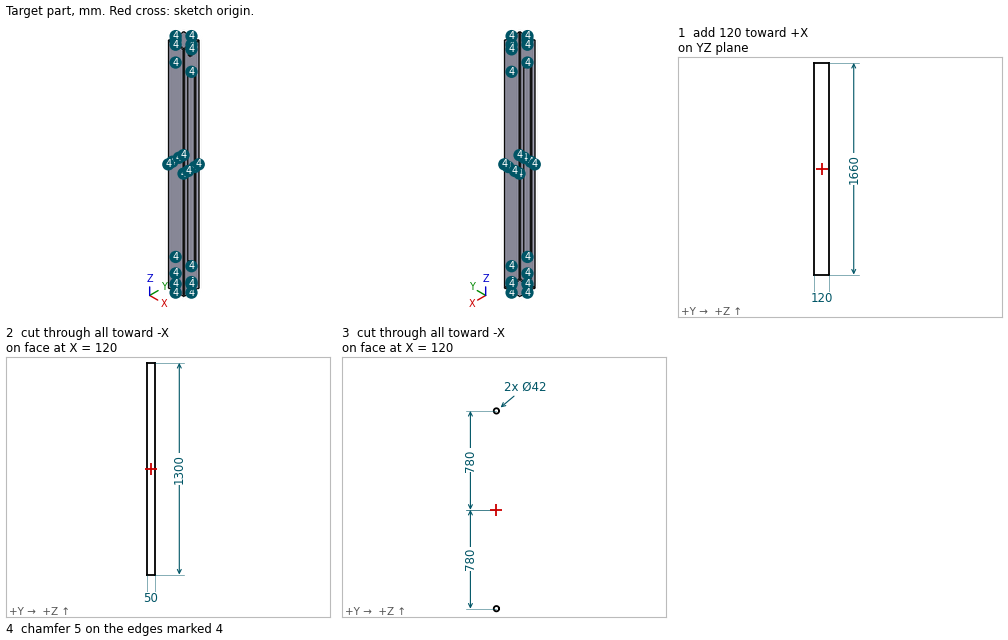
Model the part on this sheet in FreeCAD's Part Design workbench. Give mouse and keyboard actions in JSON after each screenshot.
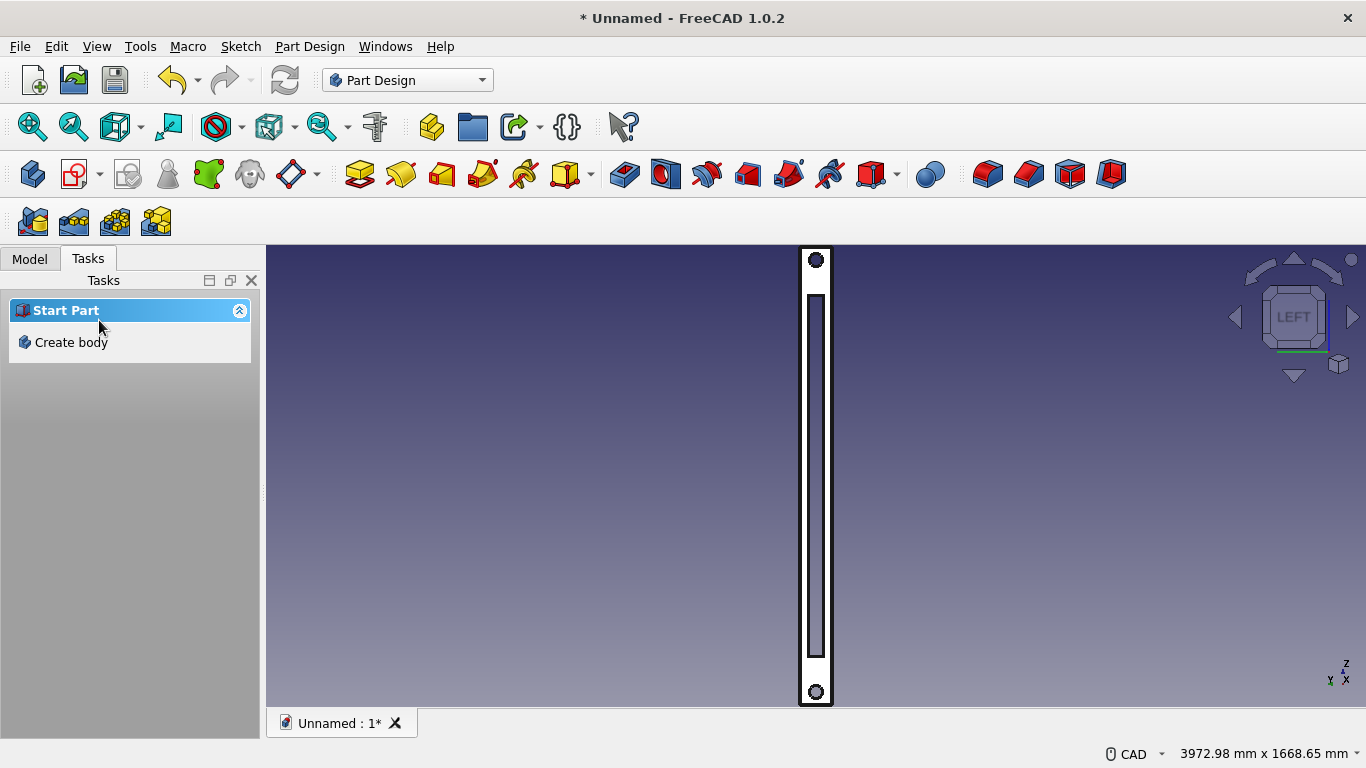
{"action": "key", "text": "0"}